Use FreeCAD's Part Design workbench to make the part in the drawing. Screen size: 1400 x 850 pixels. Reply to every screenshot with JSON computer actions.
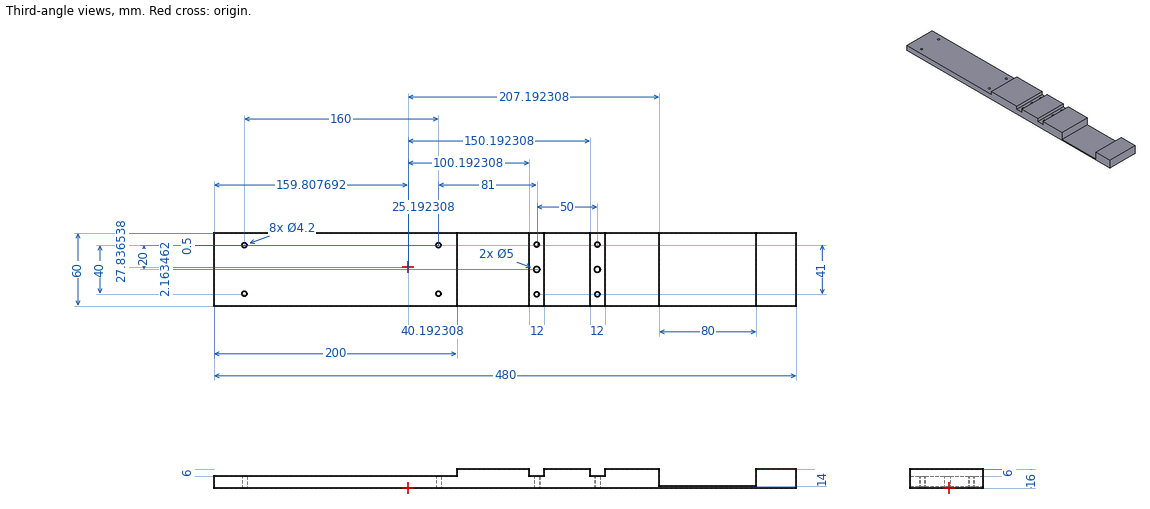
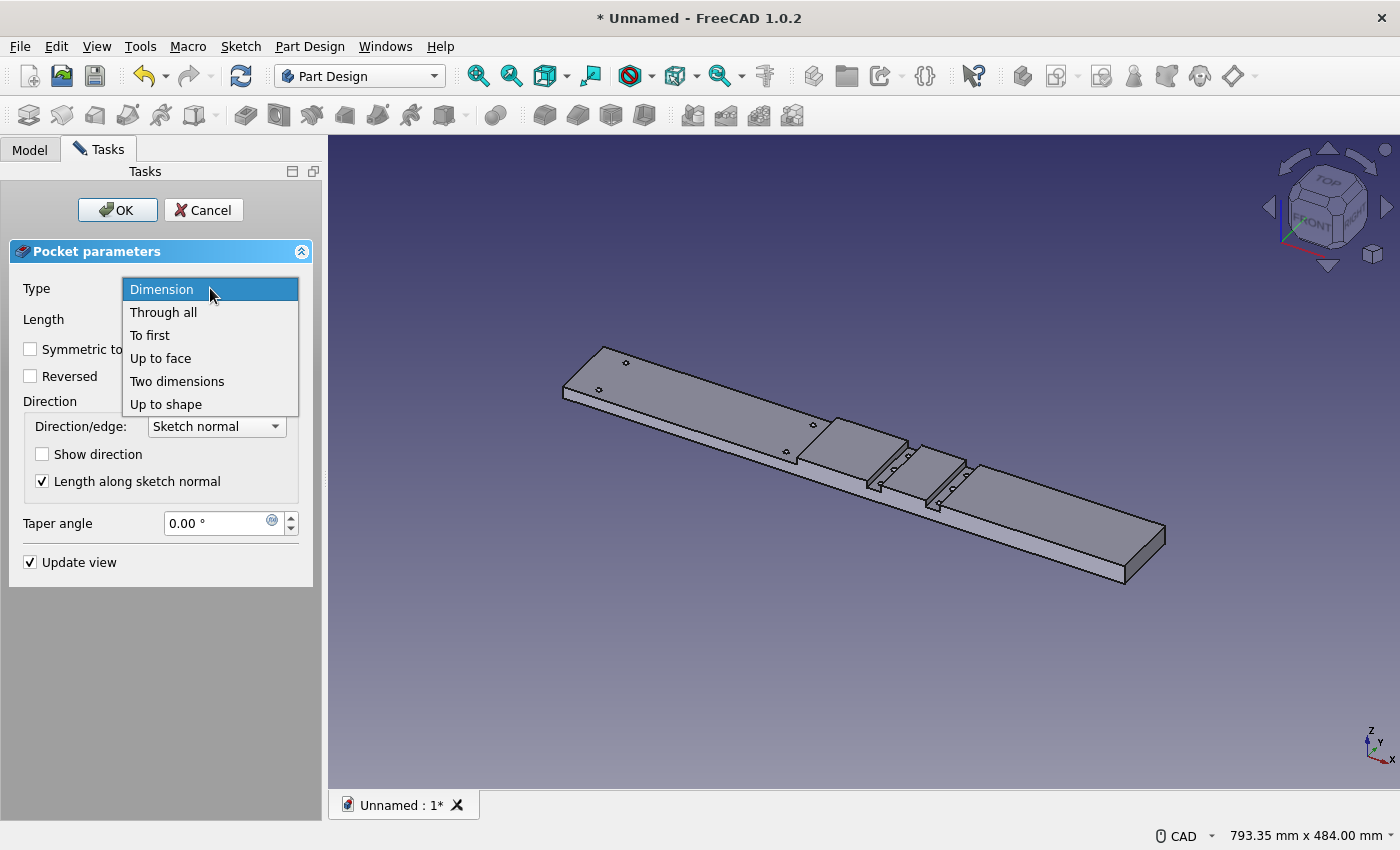
{"action": "left_click", "coordinate": [208, 312]}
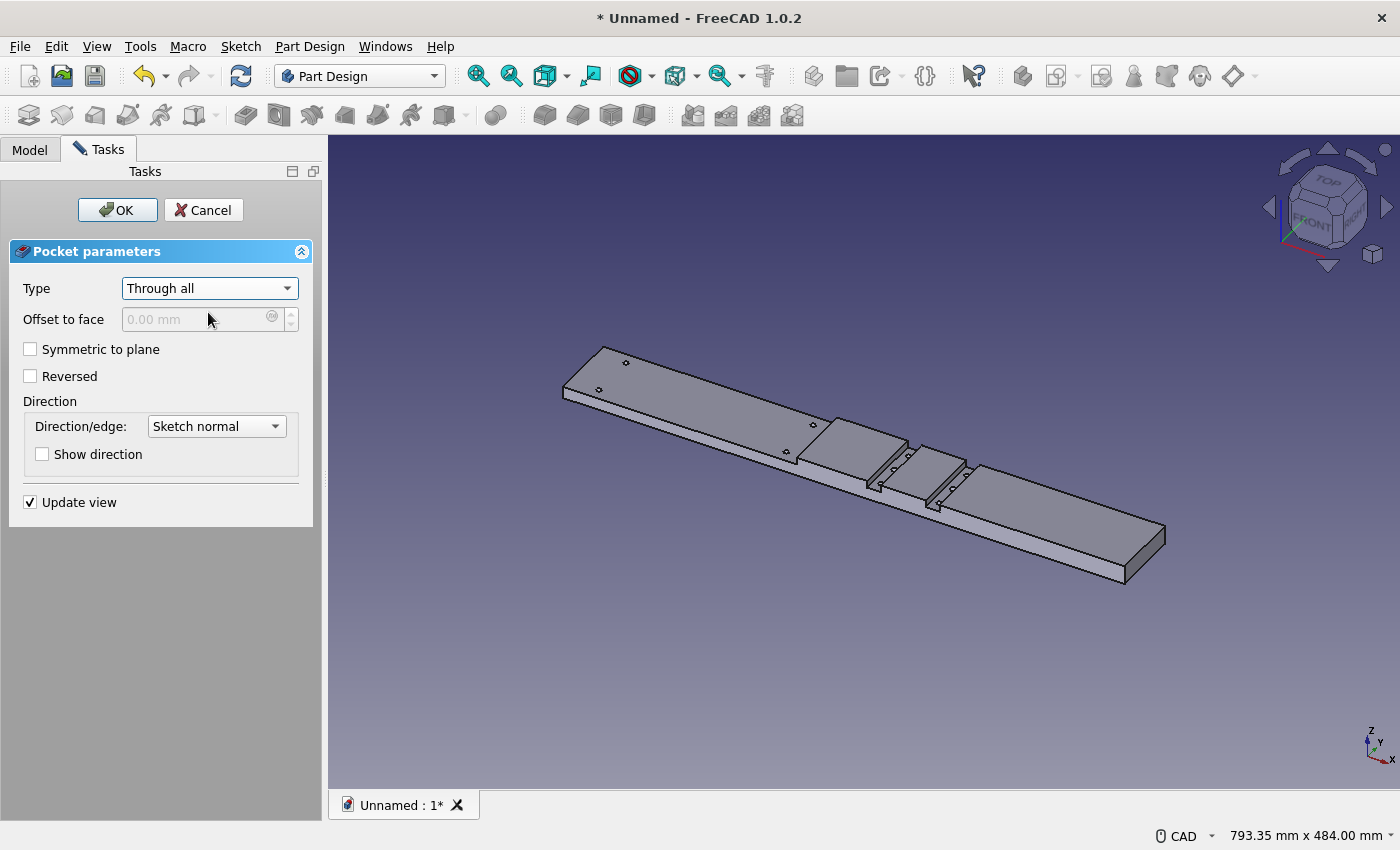
{"action": "left_click", "coordinate": [118, 210]}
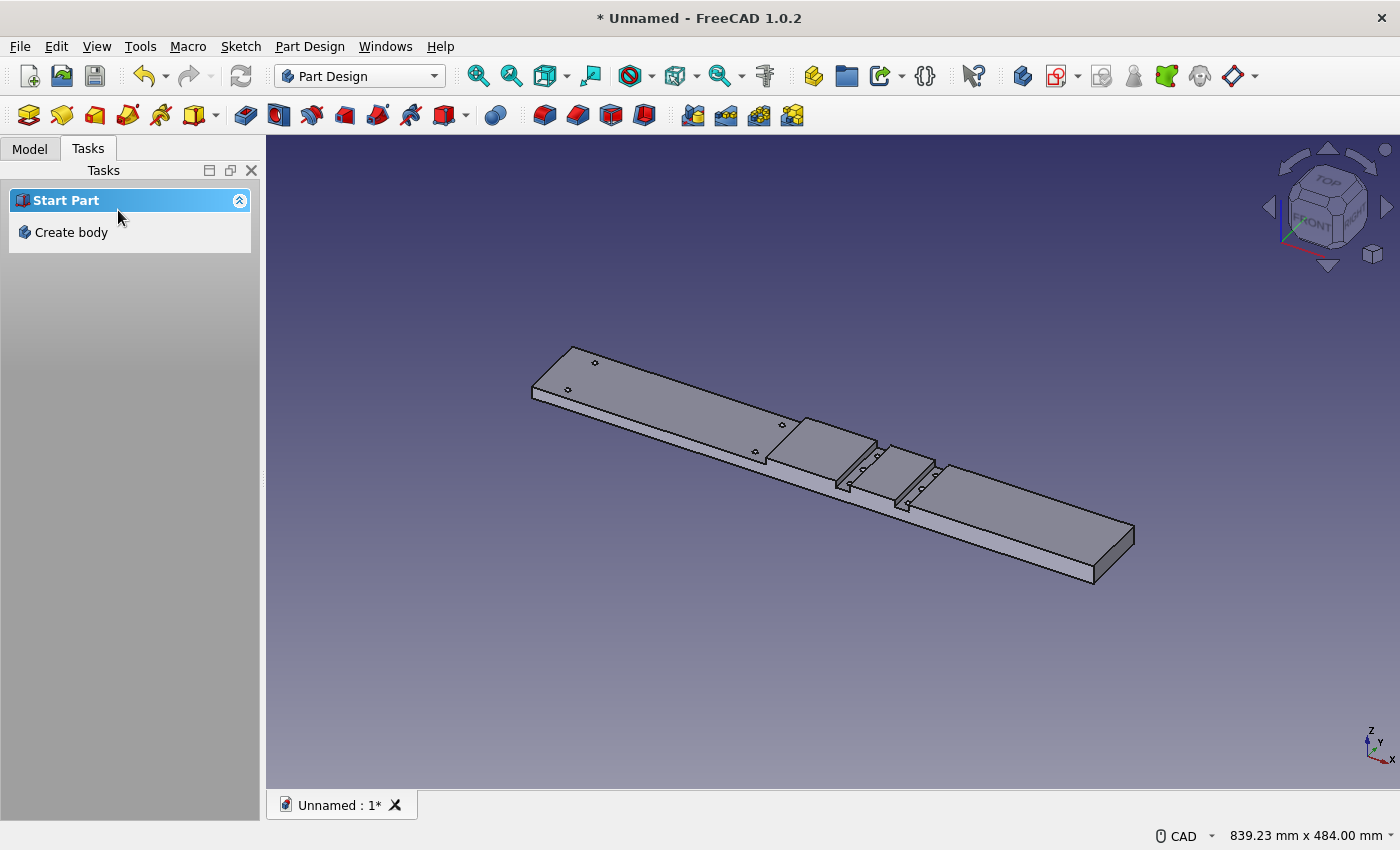
{"action": "left_click", "coordinate": [1074, 532]}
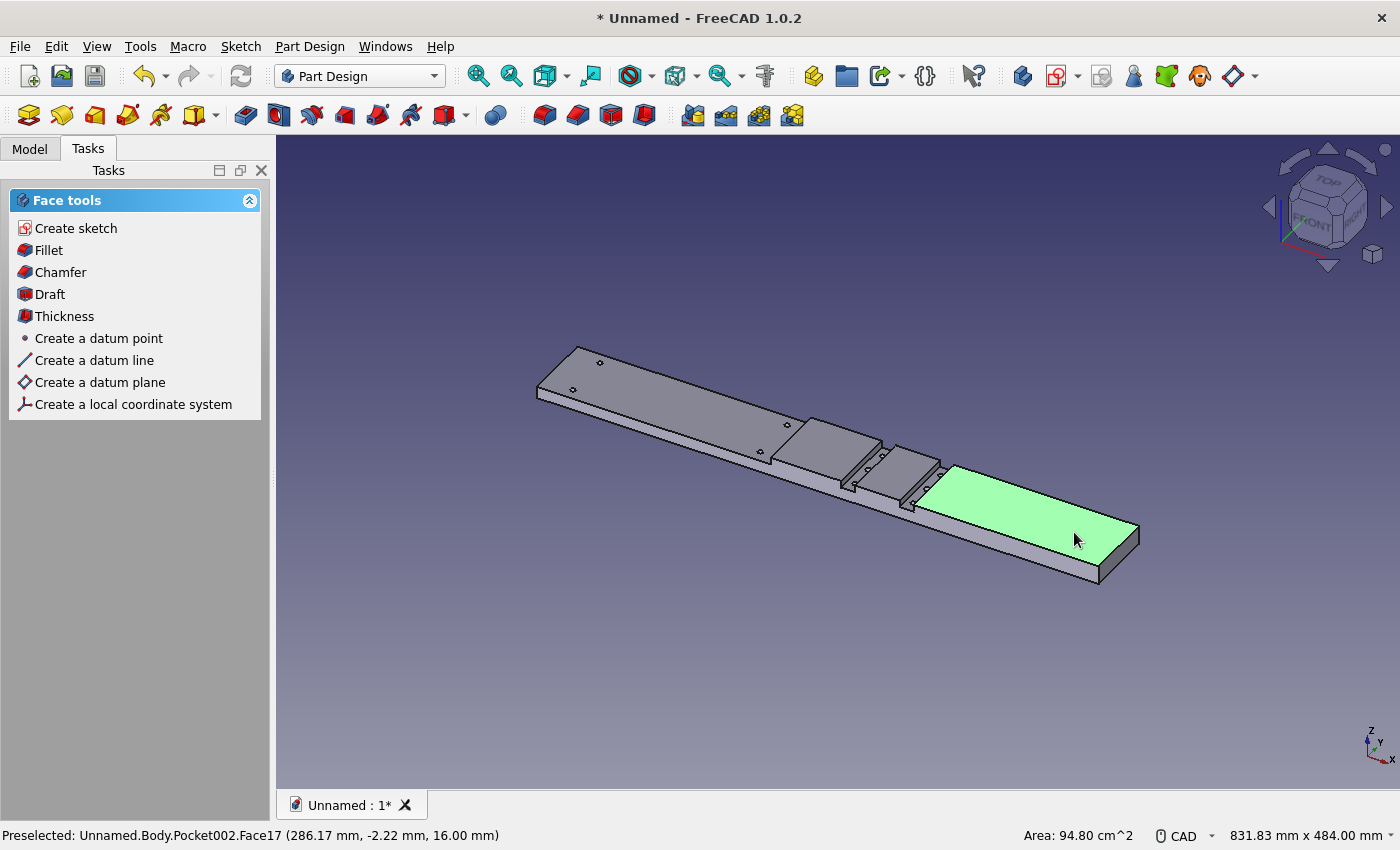
{"action": "left_click", "coordinate": [1056, 76]}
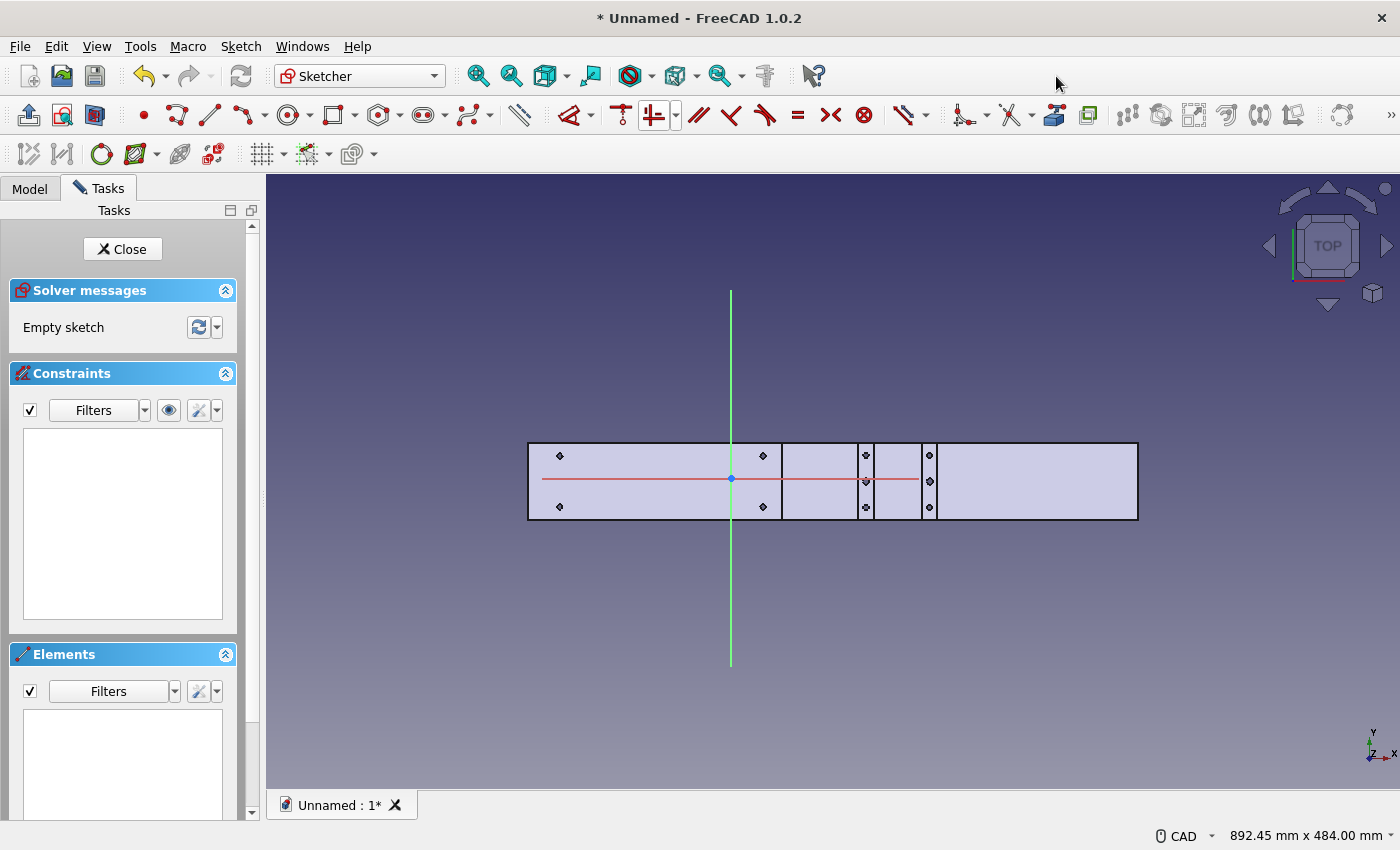
{"action": "scroll", "coordinate": [1116, 482], "scroll_direction": "up", "scroll_amount": 8}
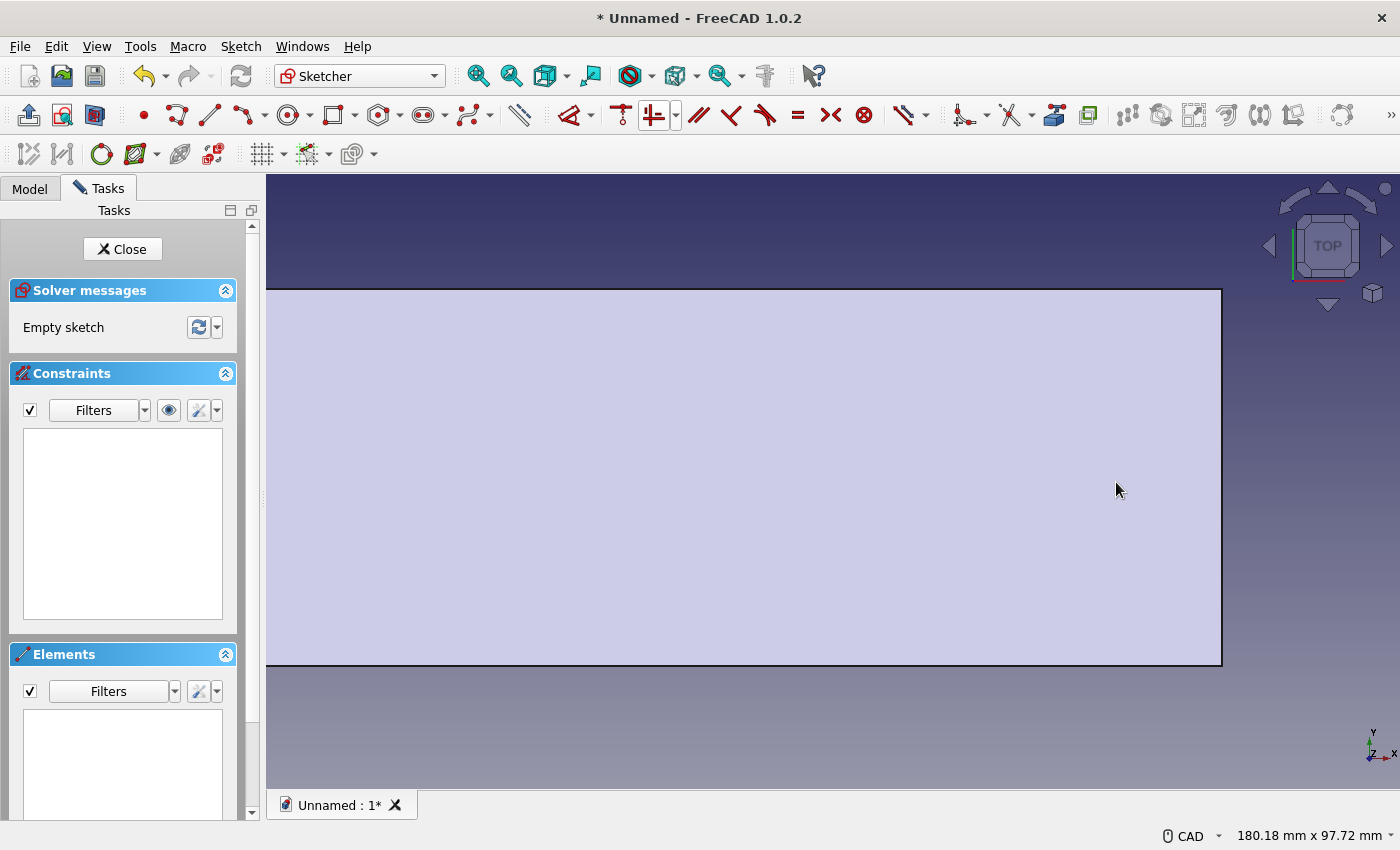
{"action": "left_click", "coordinate": [332, 116]}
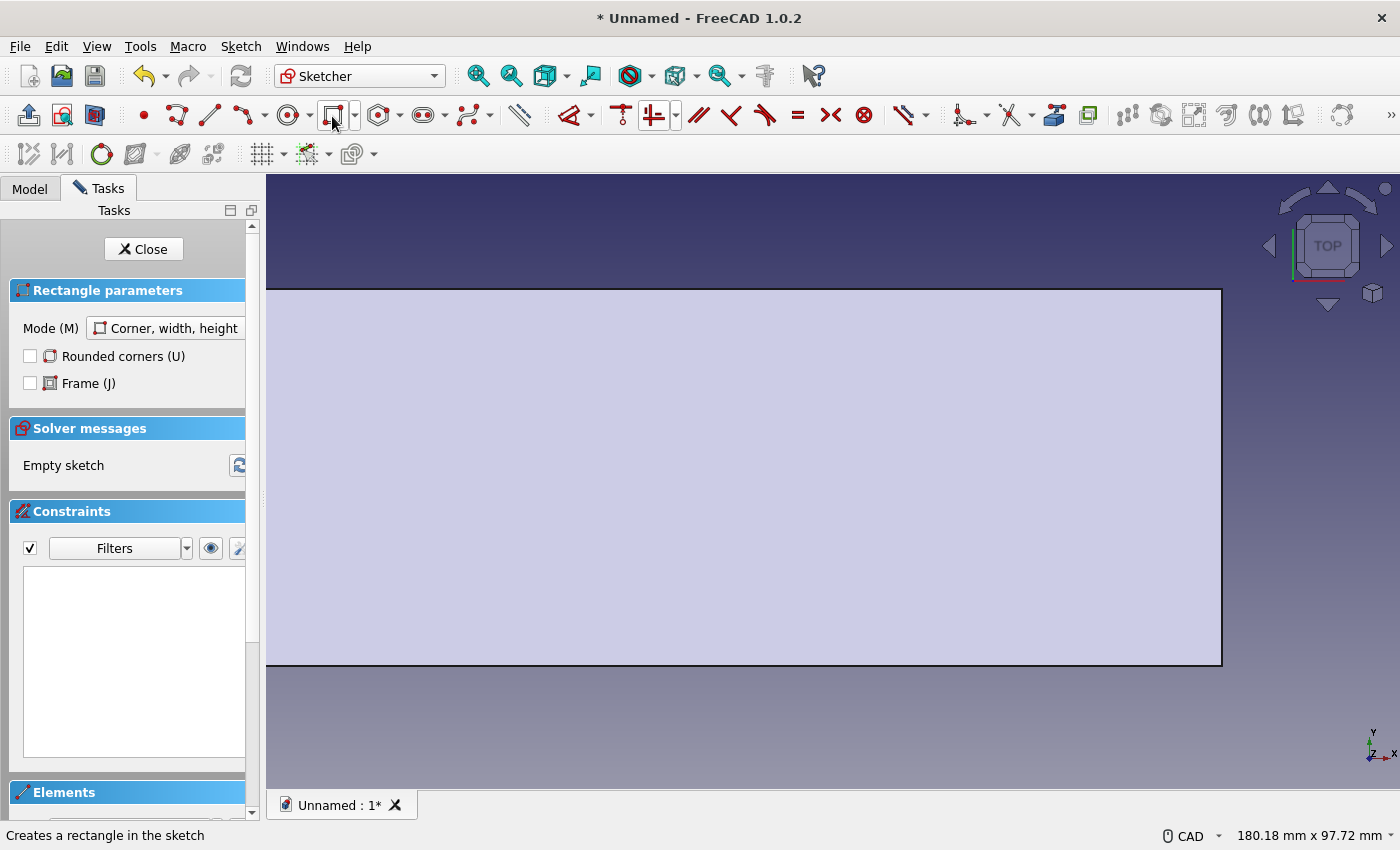
{"action": "left_click", "coordinate": [511, 289]}
{"action": "left_click", "coordinate": [1014, 666]}
{"action": "key", "text": "Escape"}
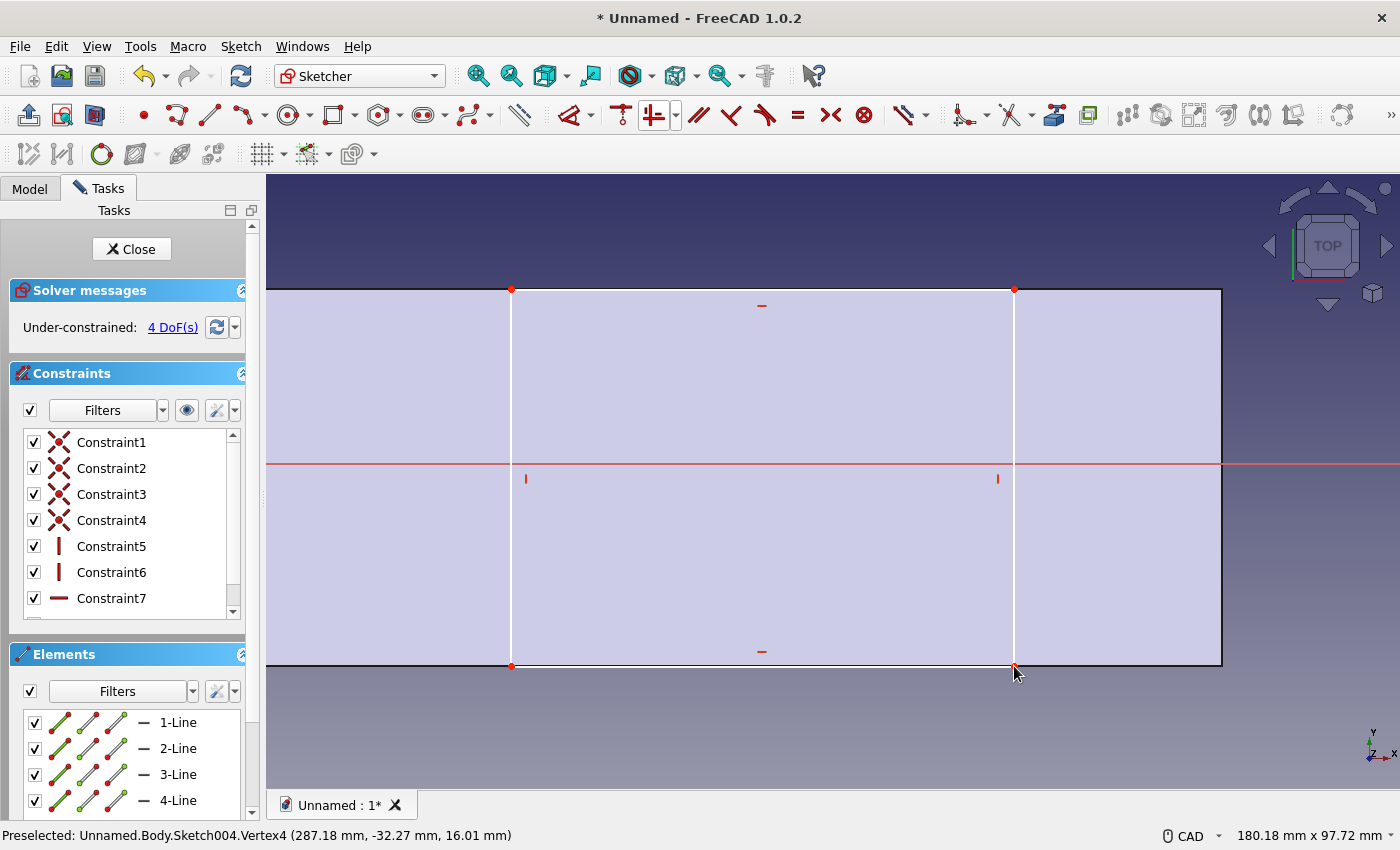
{"action": "left_click", "coordinate": [568, 116]}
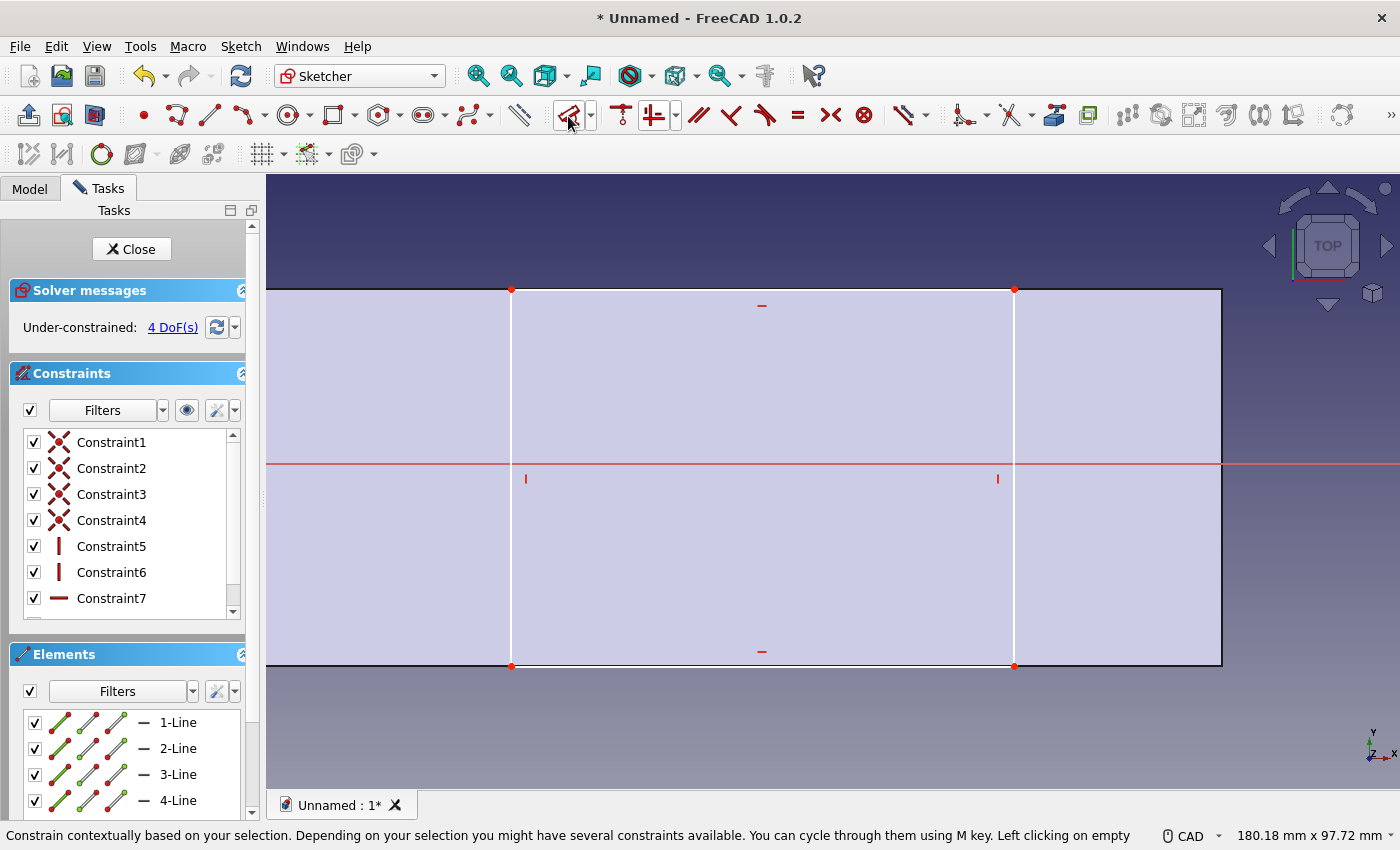
{"action": "left_click", "coordinate": [511, 403]}
{"action": "left_click", "coordinate": [477, 478]}